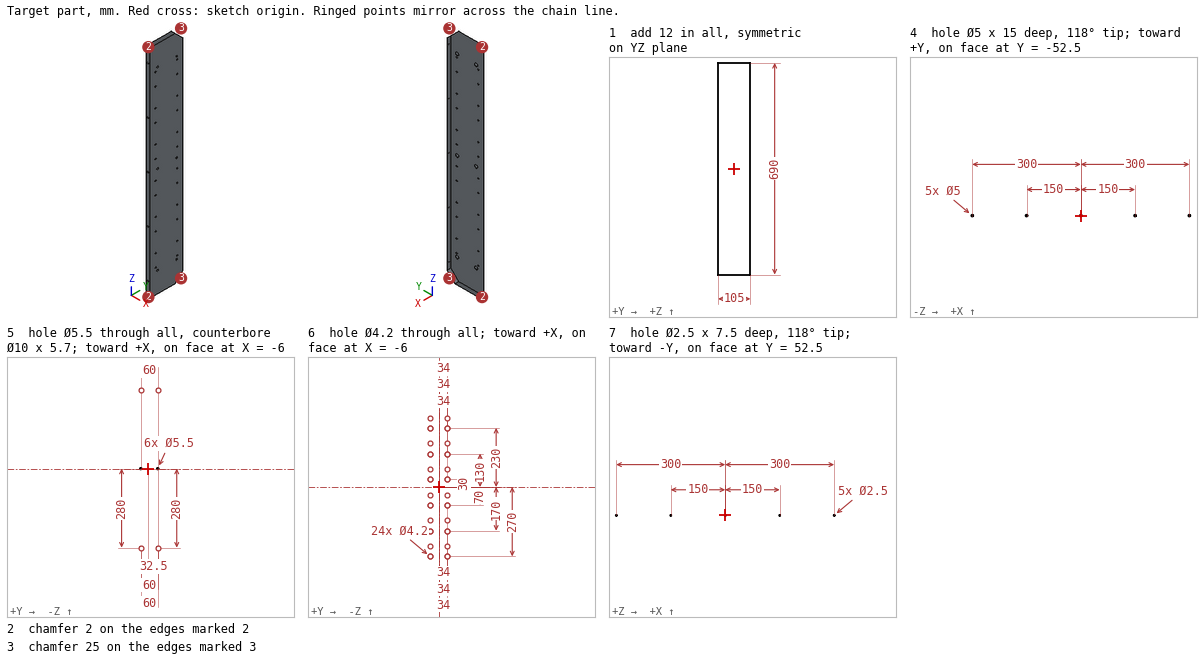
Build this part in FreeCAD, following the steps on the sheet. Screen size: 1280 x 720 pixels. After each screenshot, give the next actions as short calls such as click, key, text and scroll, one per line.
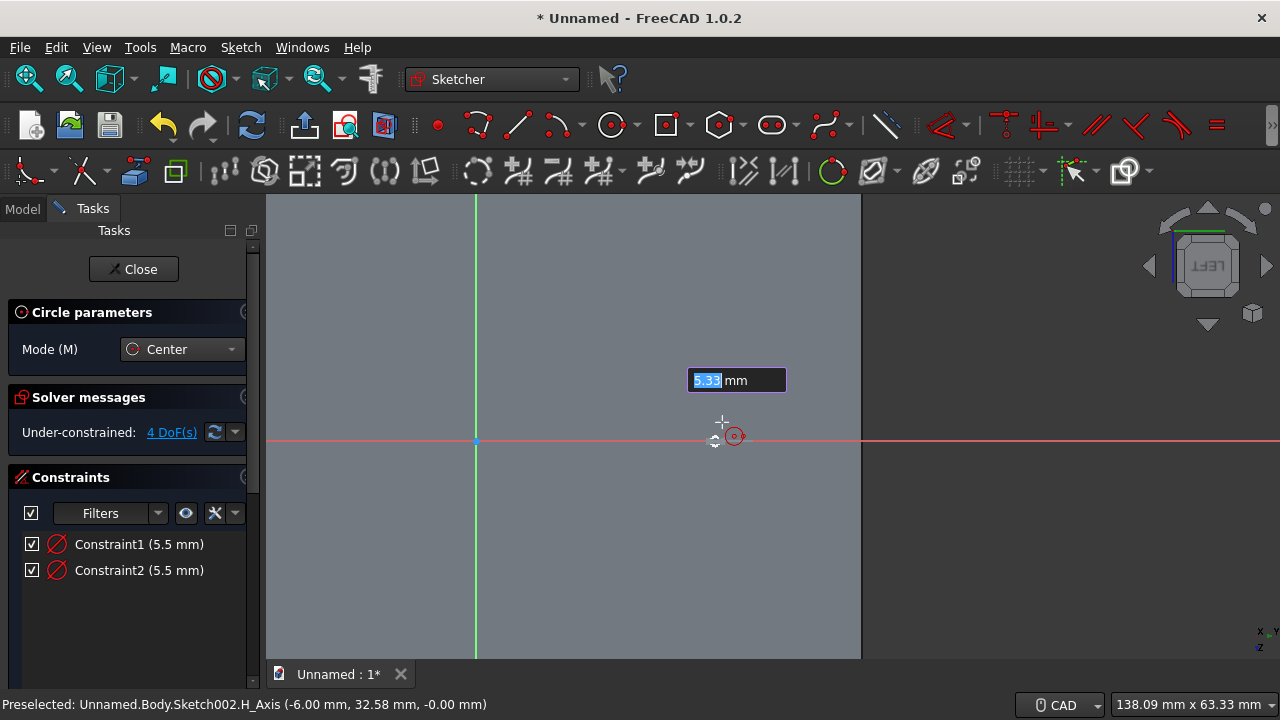
text(5.5)
key(Return)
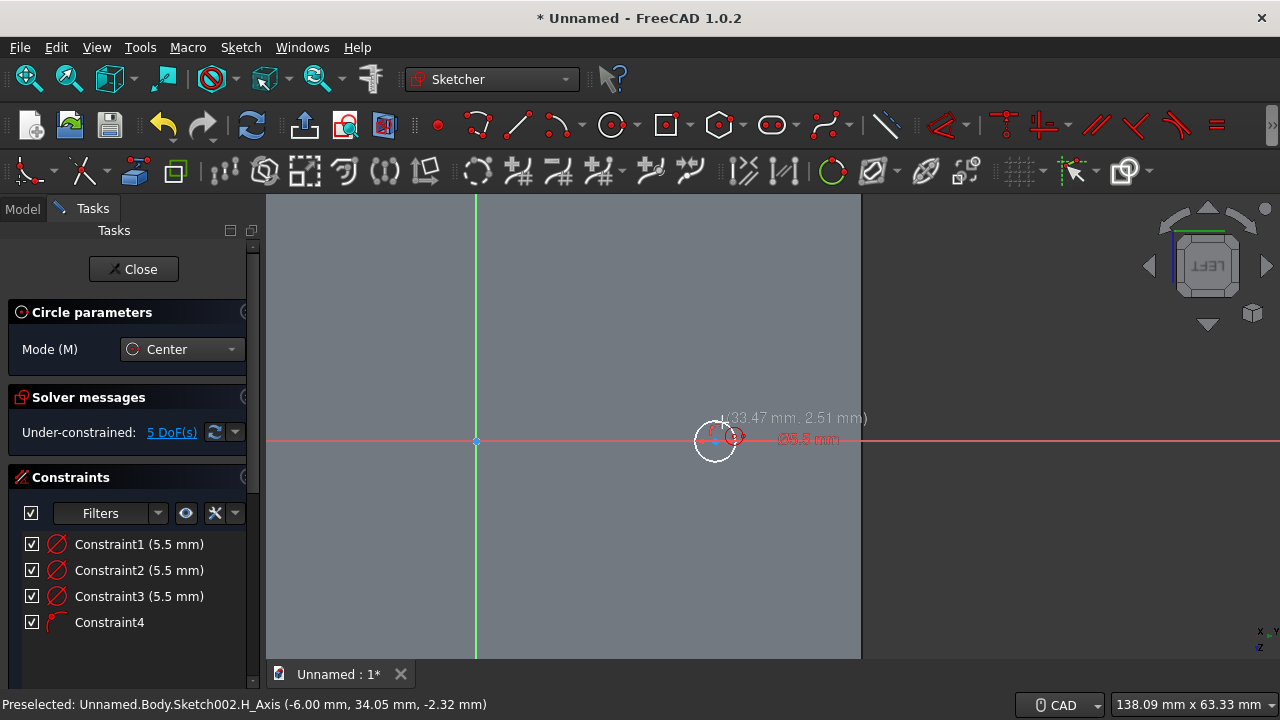
scroll(721, 425, down, 13)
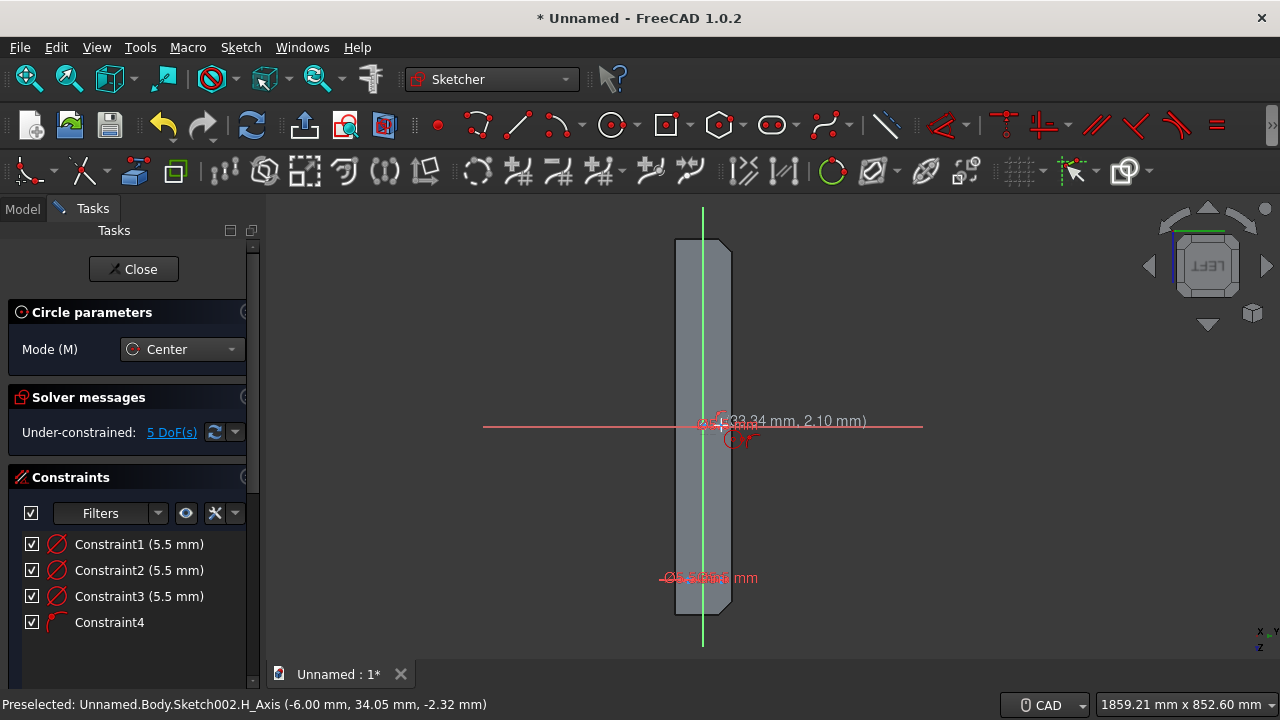
scroll(688, 427, up, 14)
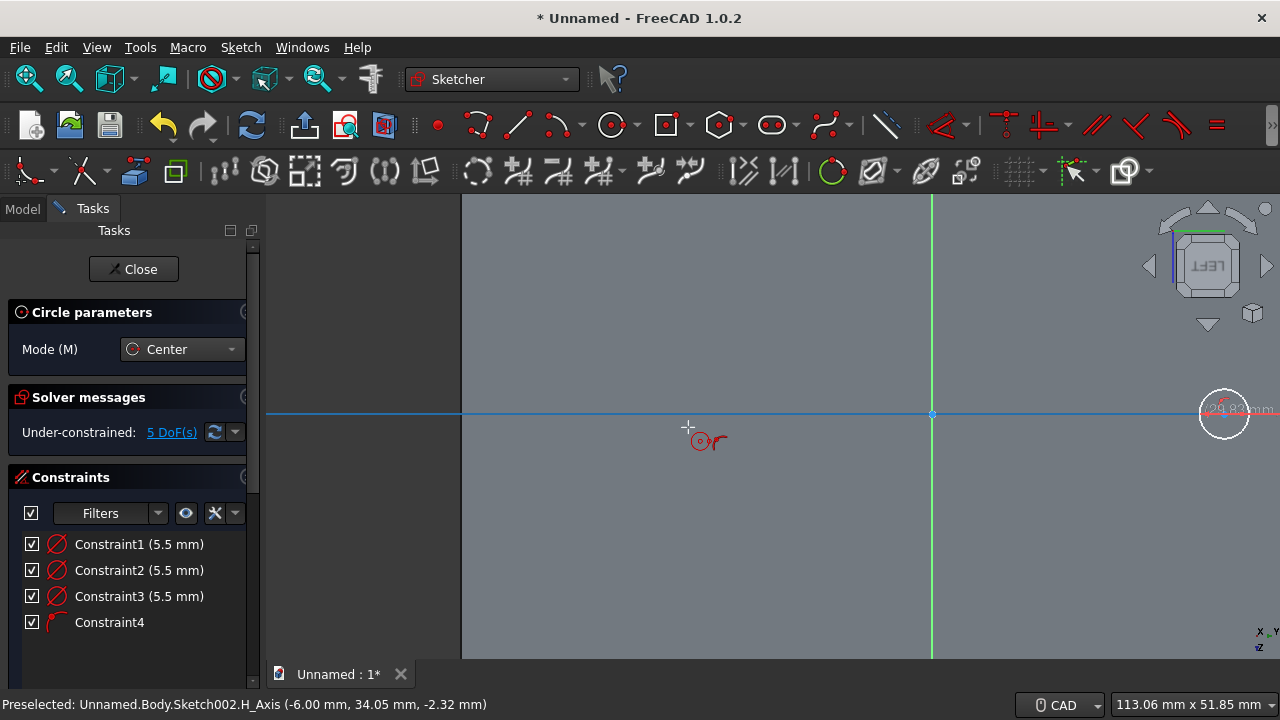
scroll(688, 427, down, 14)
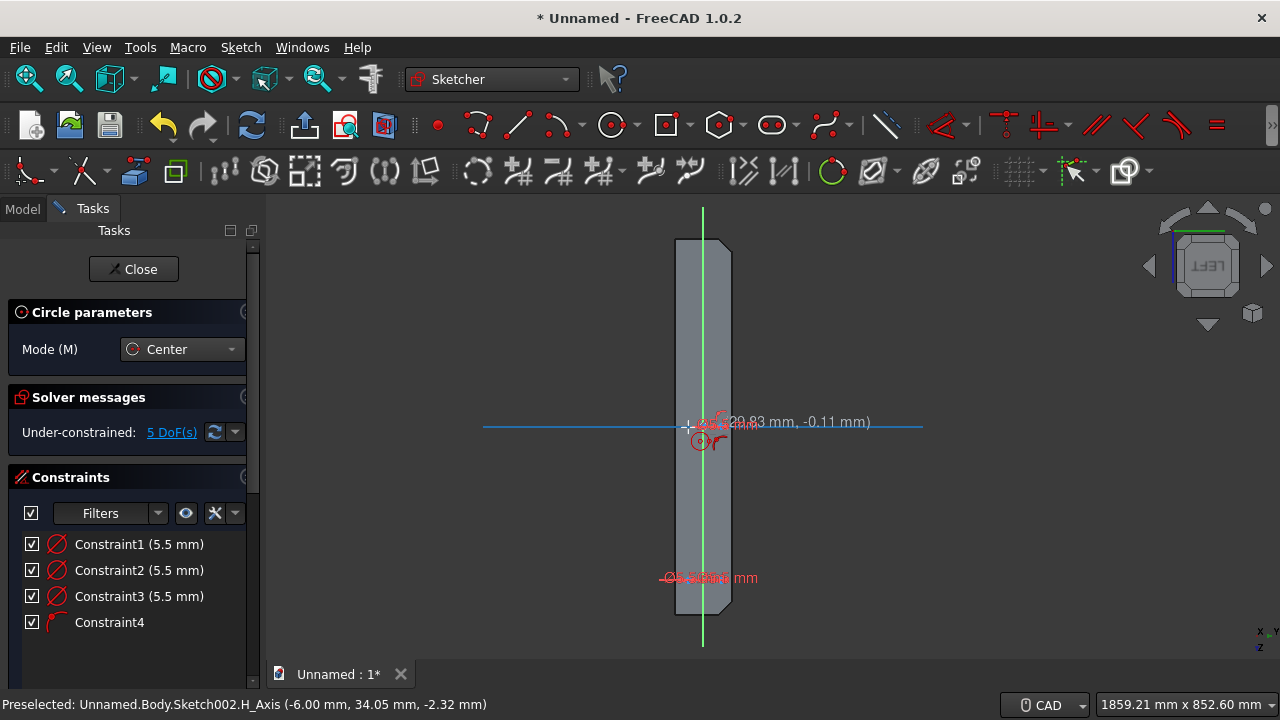
click(688, 427)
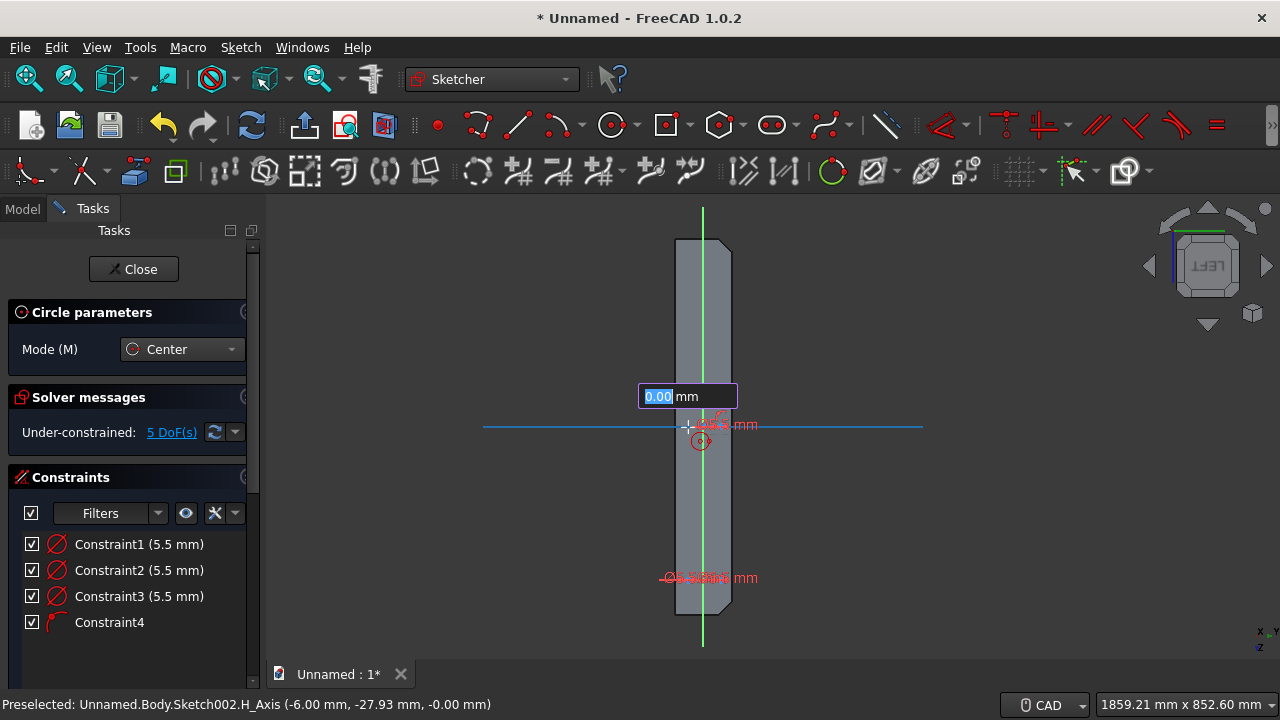
scroll(689, 425, up, 13)
move(680, 422)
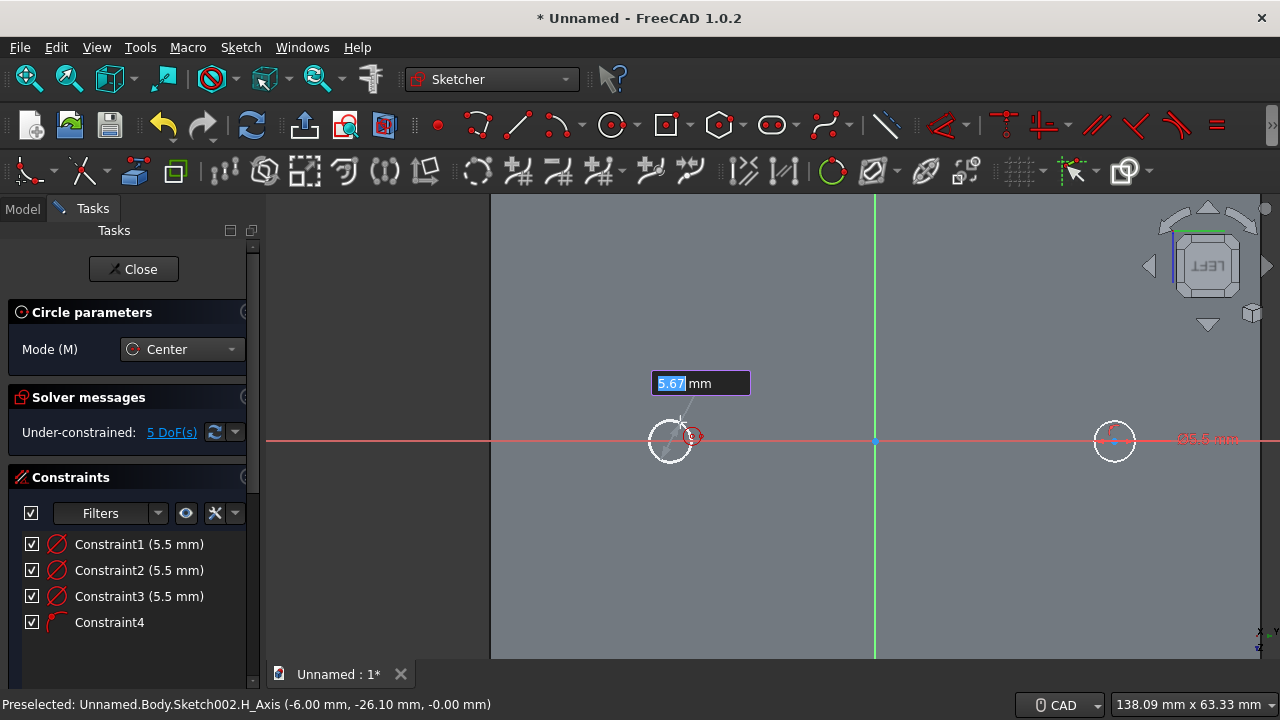
text(5.5)
key(Return)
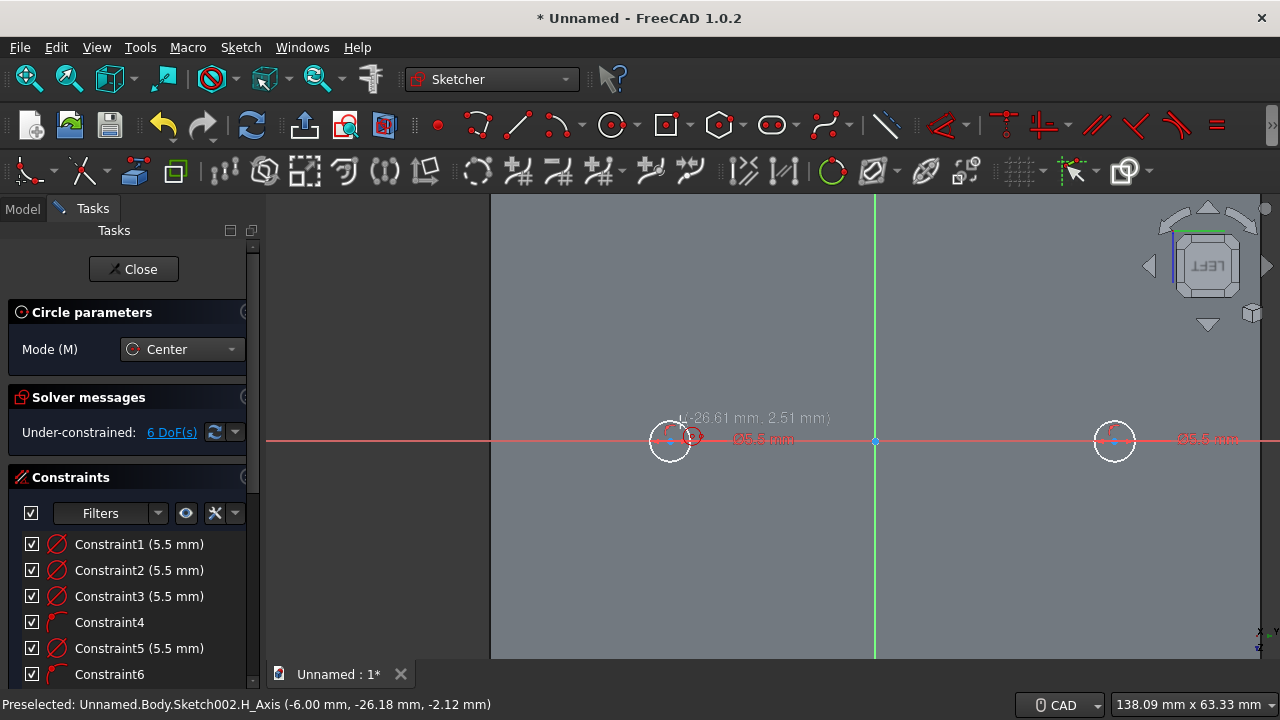
scroll(689, 425, down, 13)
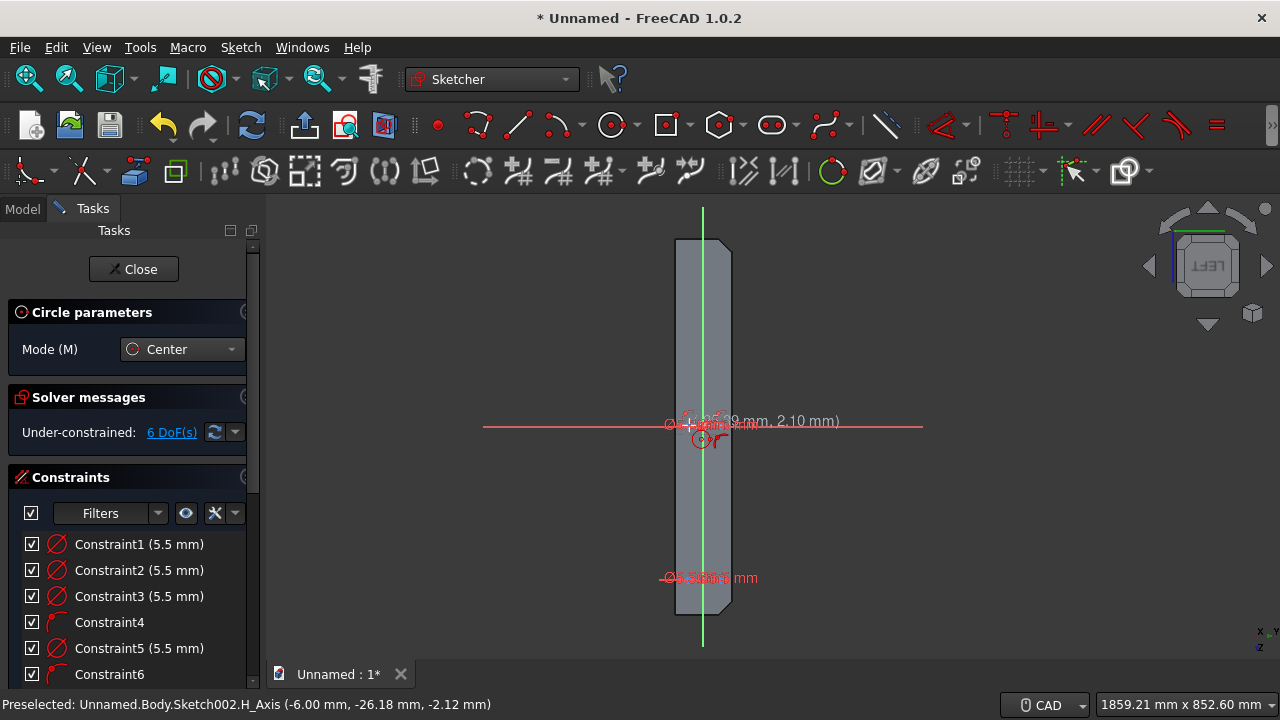
scroll(721, 274, up, 14)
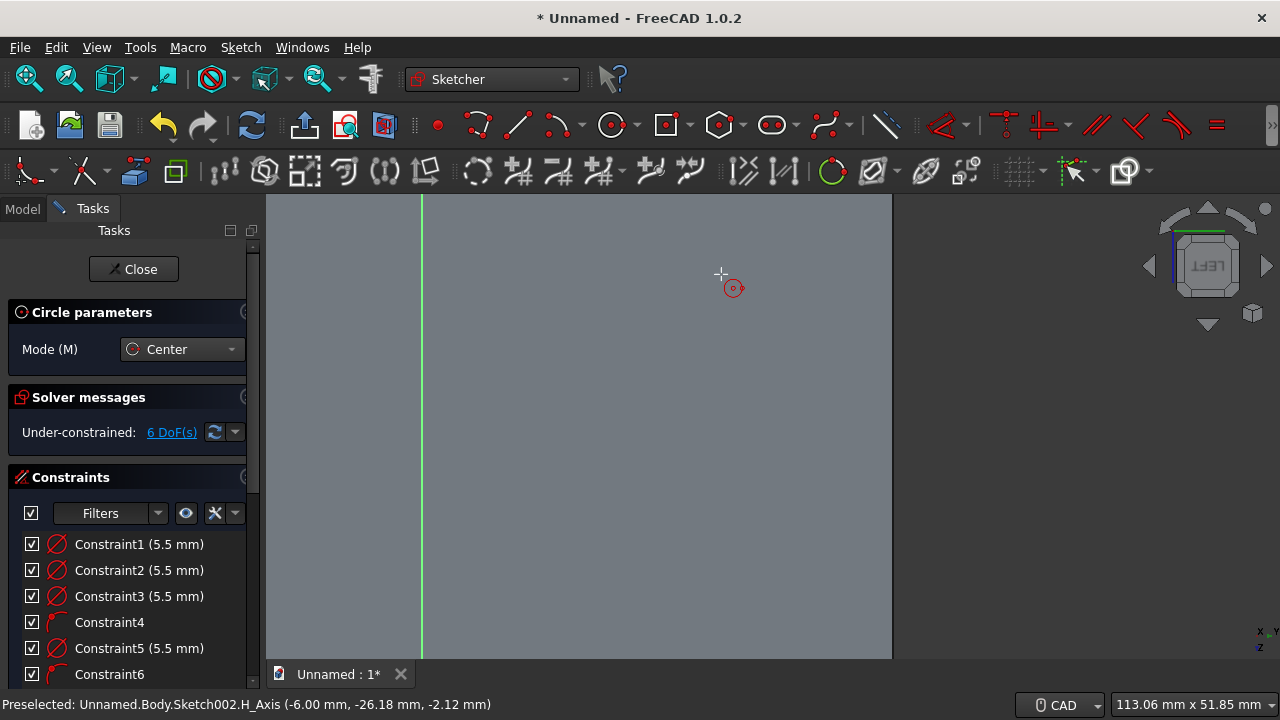
scroll(721, 274, down, 14)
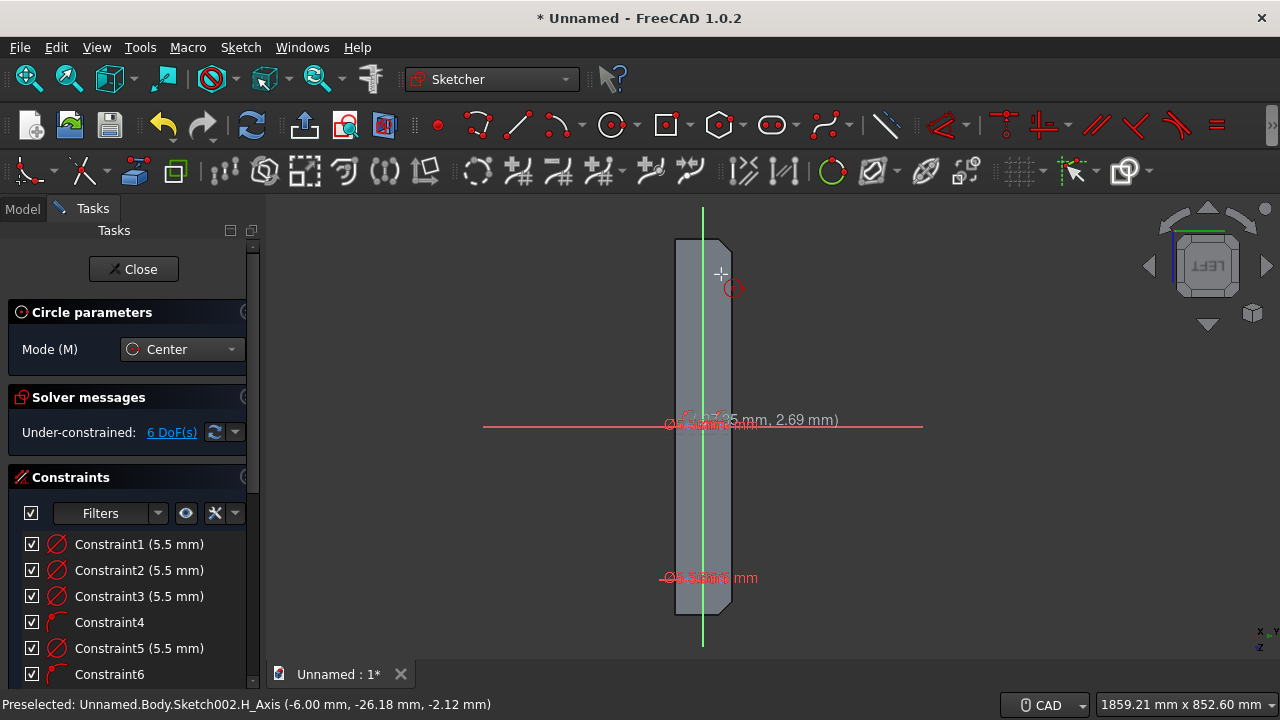
click(721, 274)
move(722, 273)